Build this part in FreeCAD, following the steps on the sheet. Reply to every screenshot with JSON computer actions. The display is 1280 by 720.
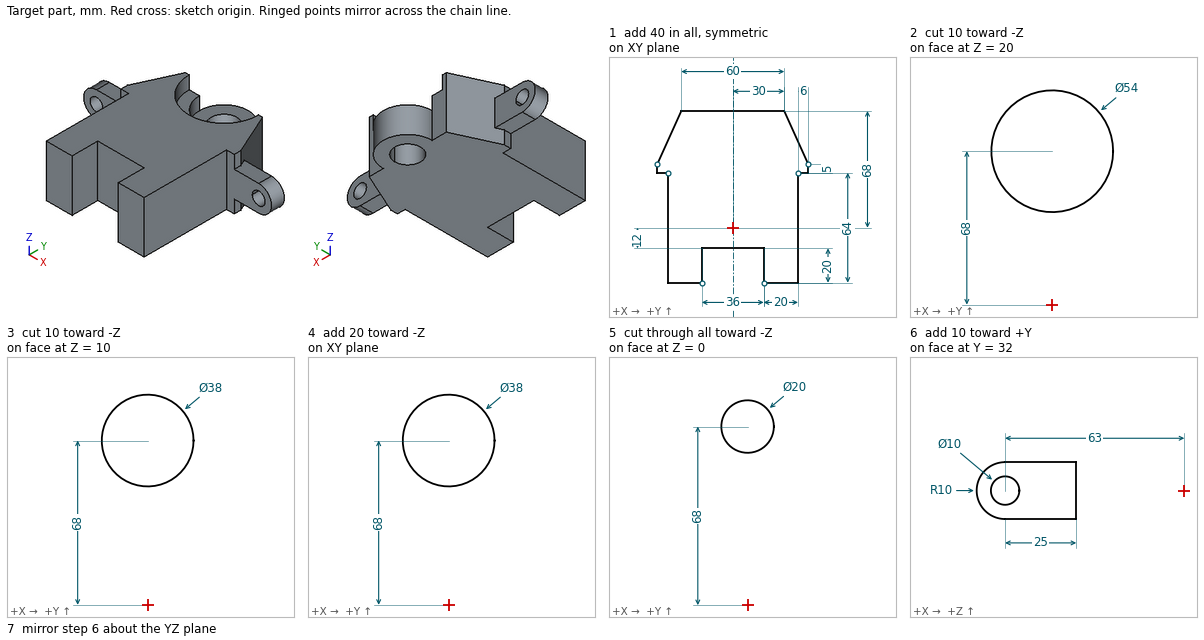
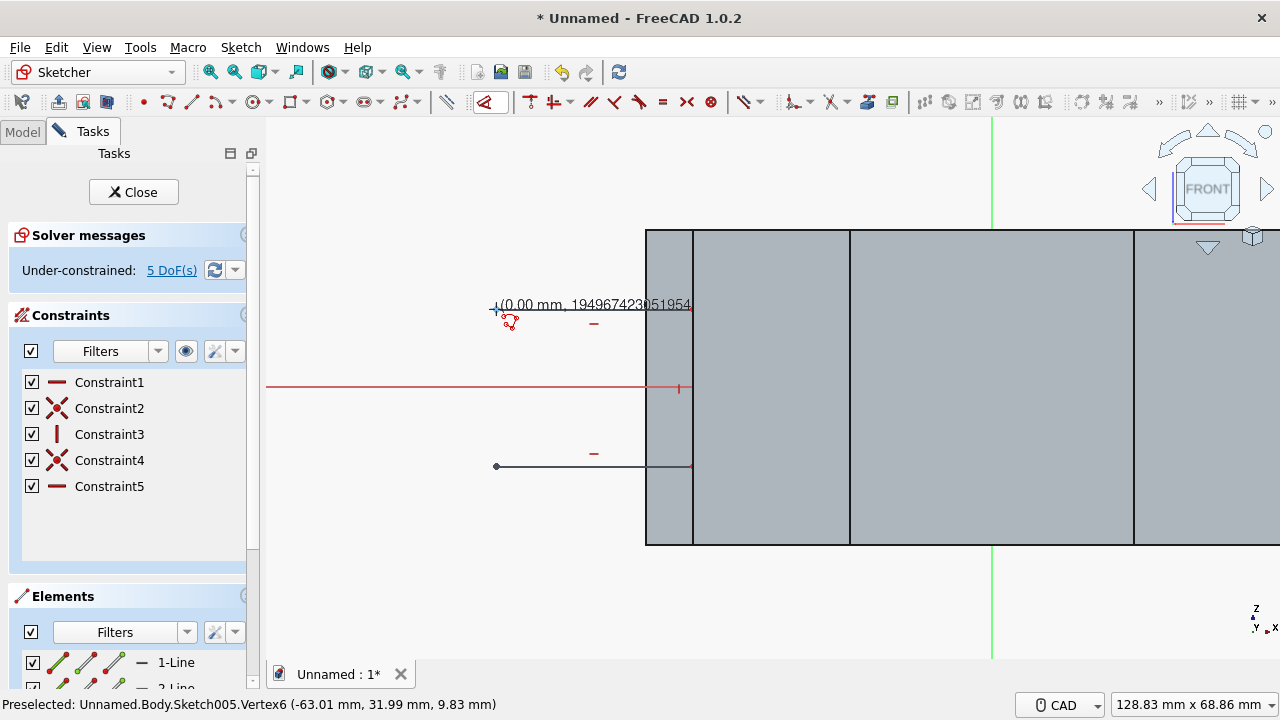
{"action": "key", "text": "g 3 a"}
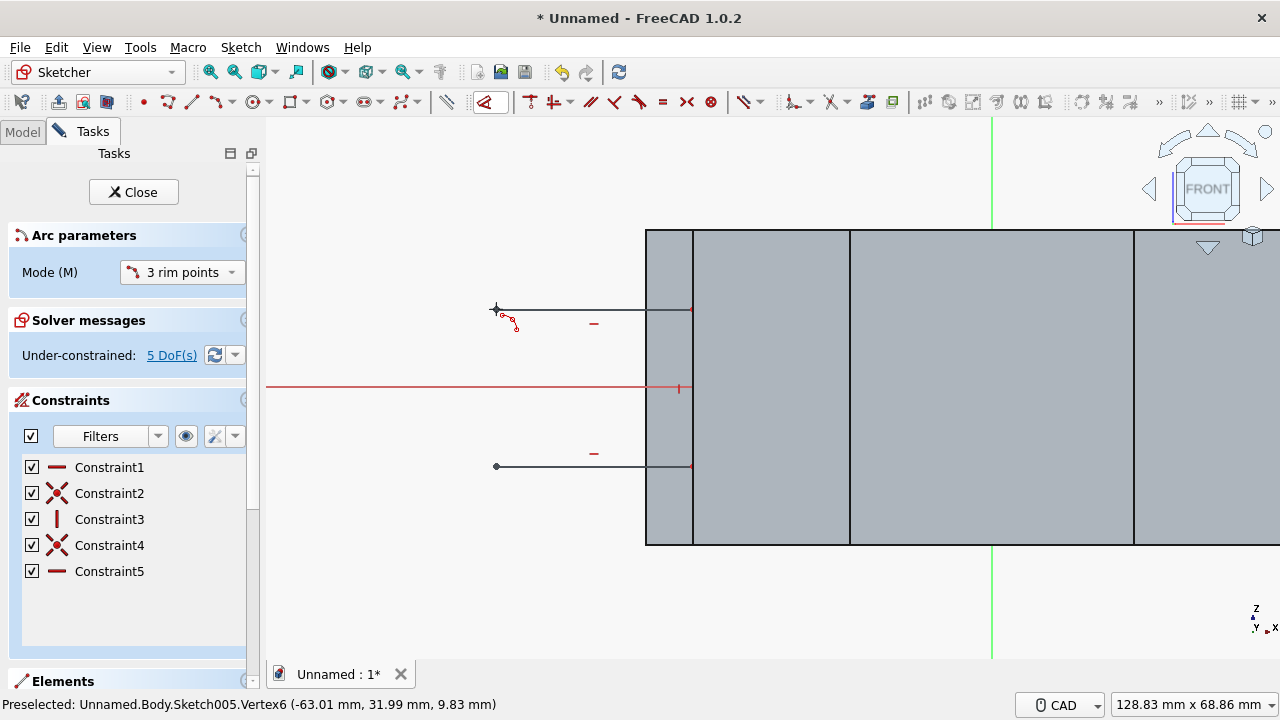
{"action": "left_click", "coordinate": [496, 310]}
{"action": "left_click", "coordinate": [496, 467]}
{"action": "left_click", "coordinate": [421, 363]}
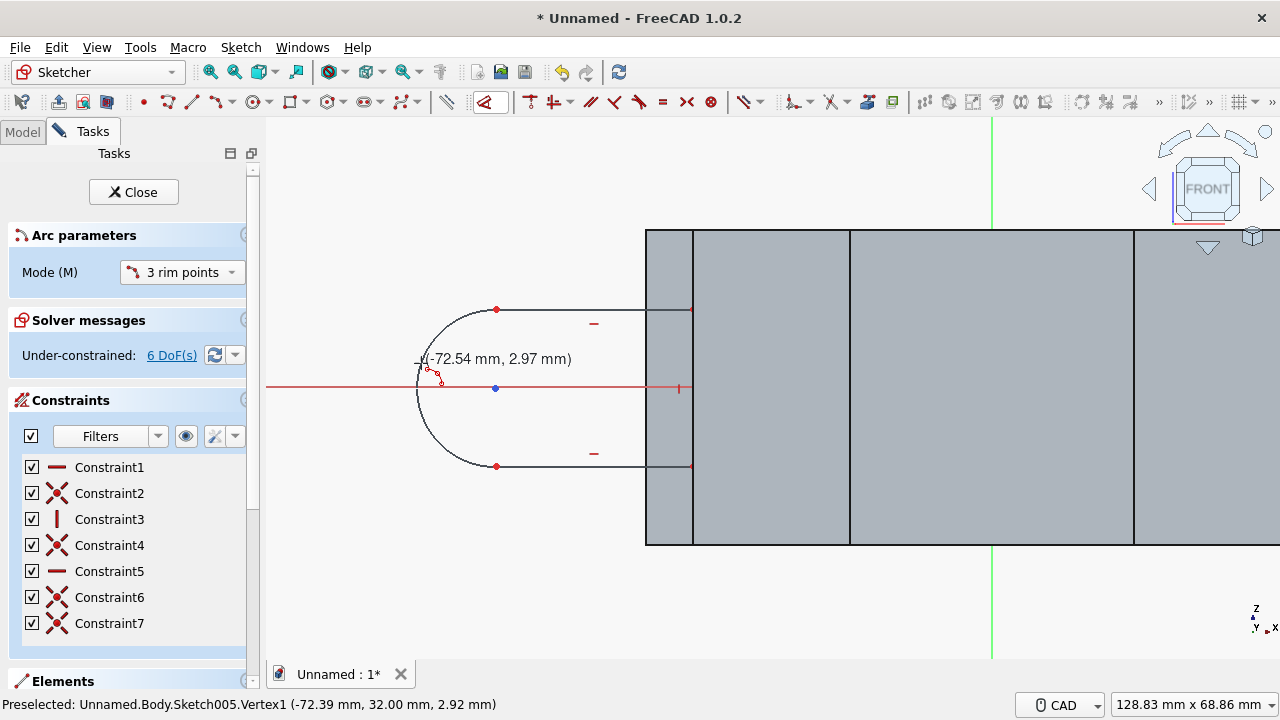
{"action": "left_click", "coordinate": [254, 102]}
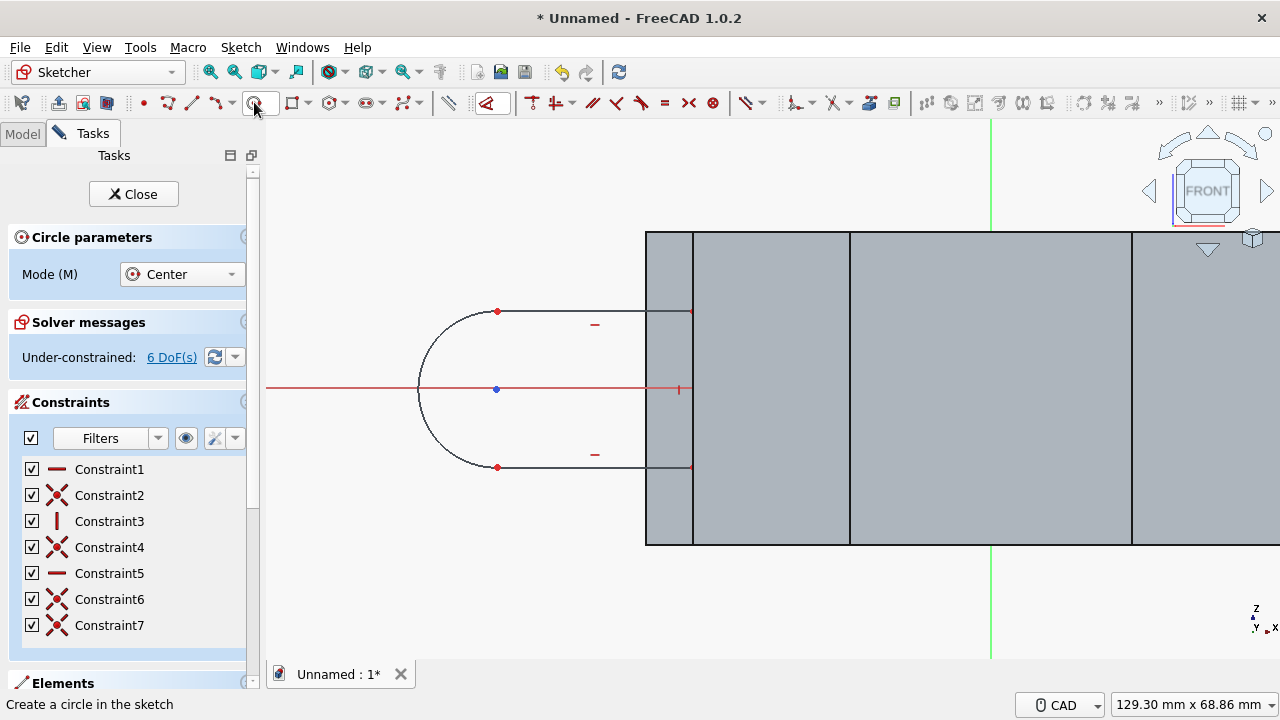
{"action": "left_click", "coordinate": [497, 388]}
{"action": "left_click", "coordinate": [525, 361]}
{"action": "key", "text": "Escape"}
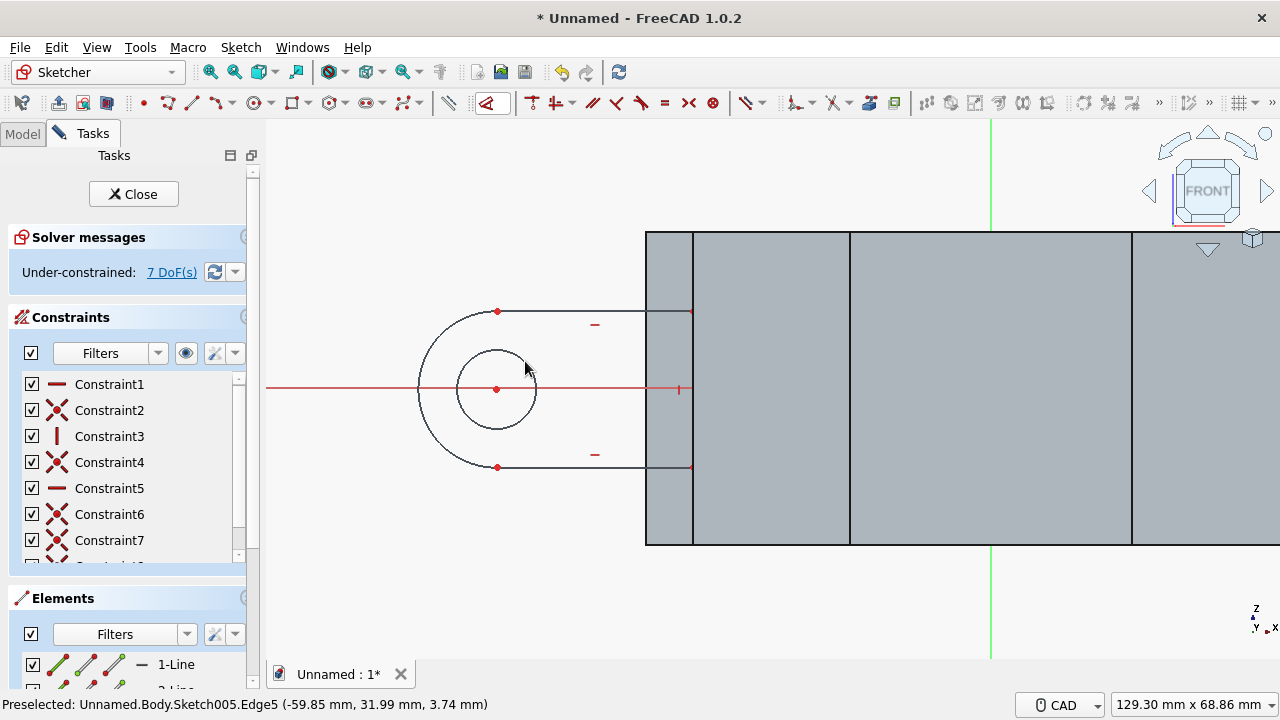
{"action": "left_click", "coordinate": [556, 468]}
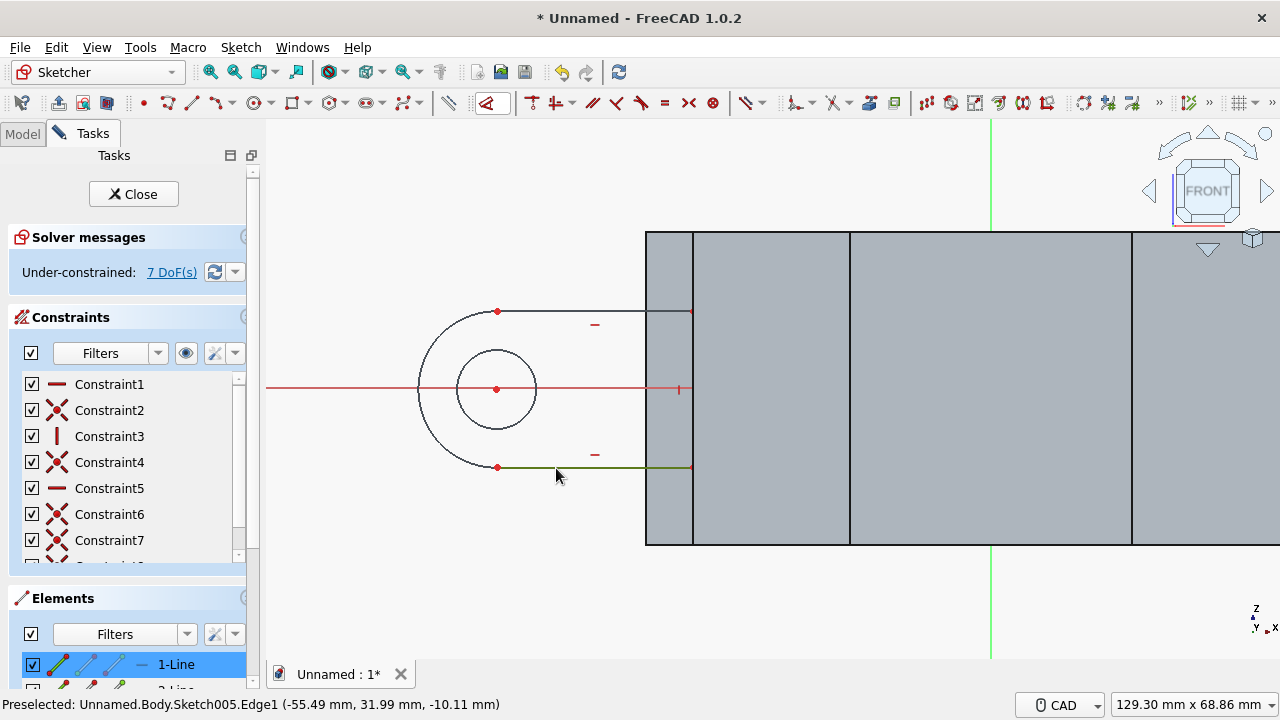
{"action": "left_click", "coordinate": [433, 343]}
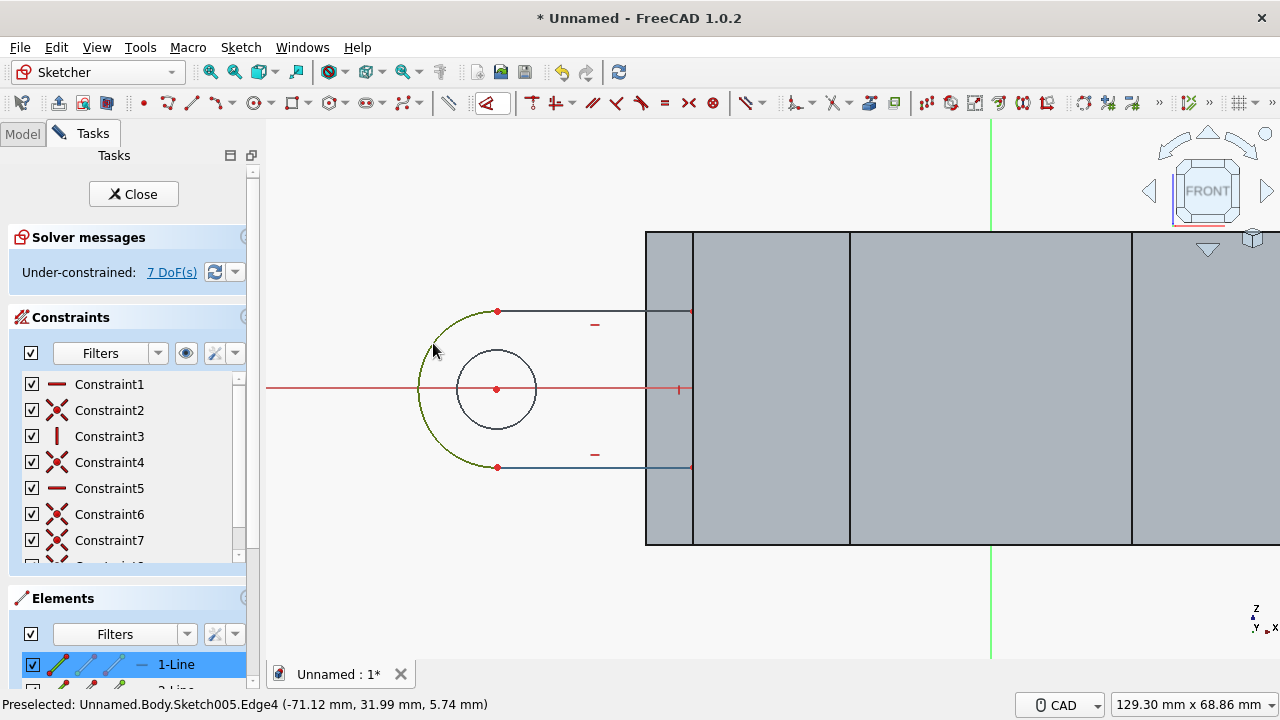
{"action": "left_click", "coordinate": [642, 104]}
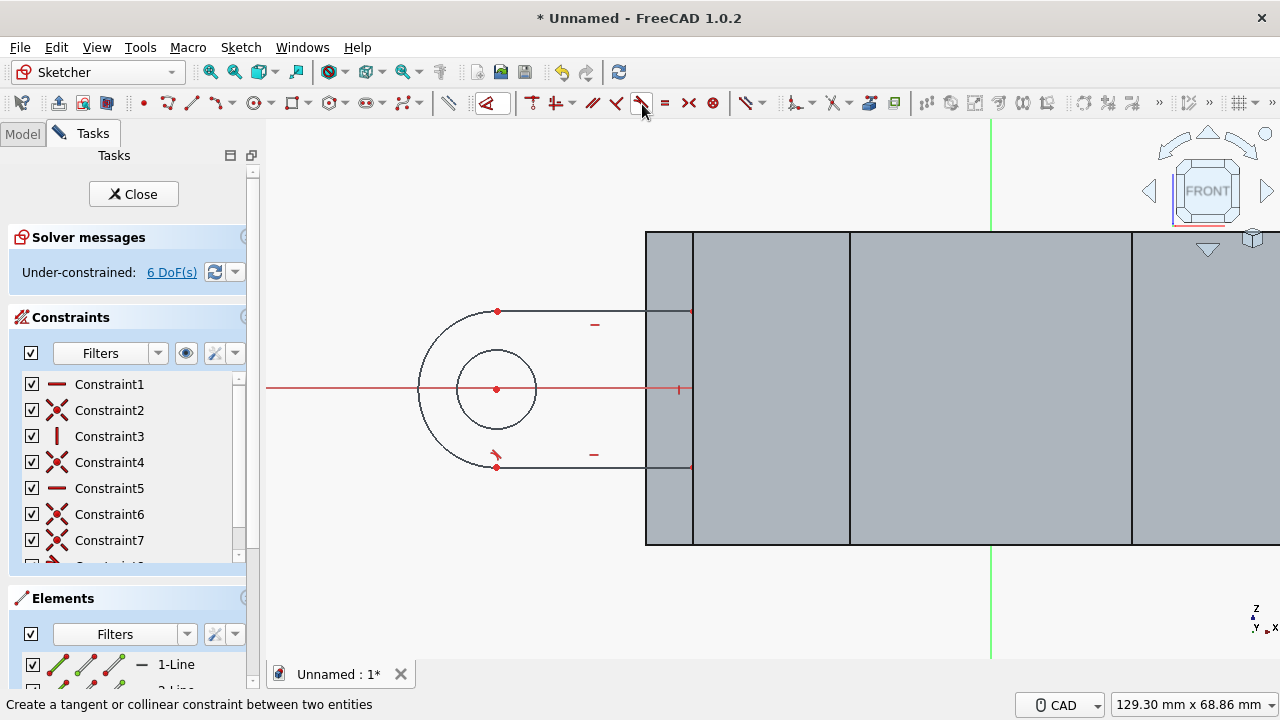
{"action": "left_click", "coordinate": [634, 311]}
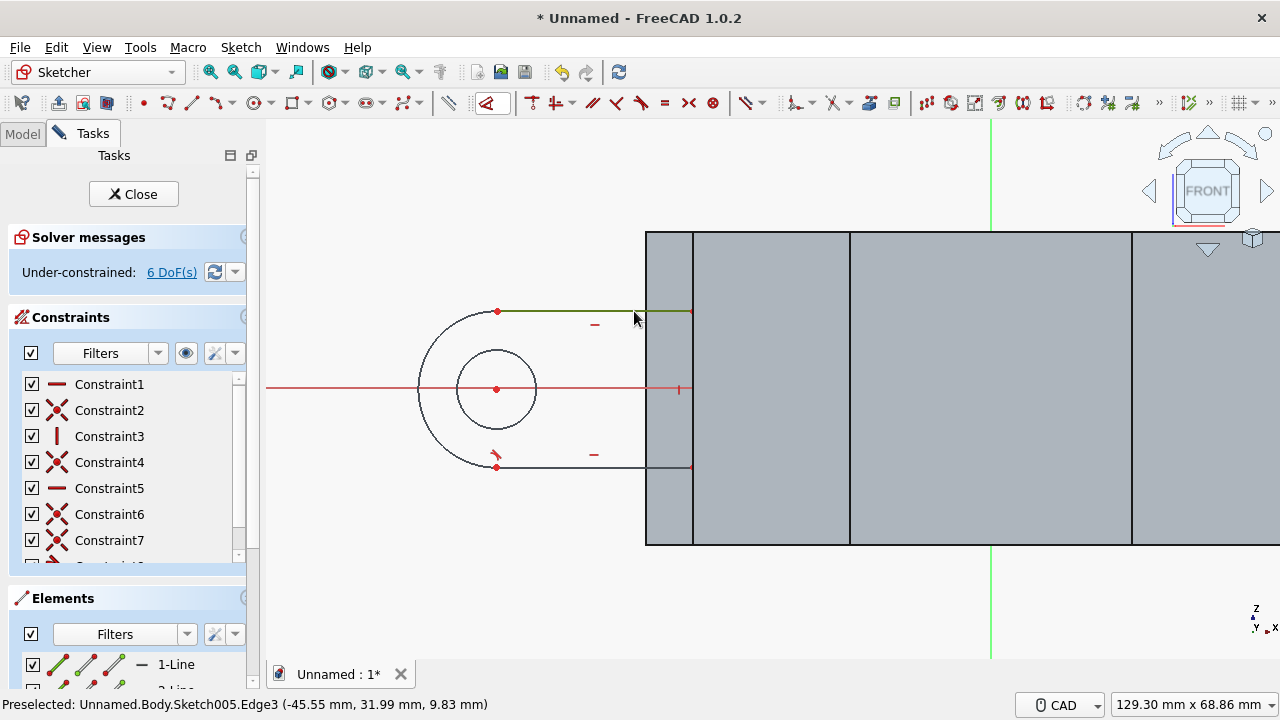
{"action": "left_click", "coordinate": [434, 343]}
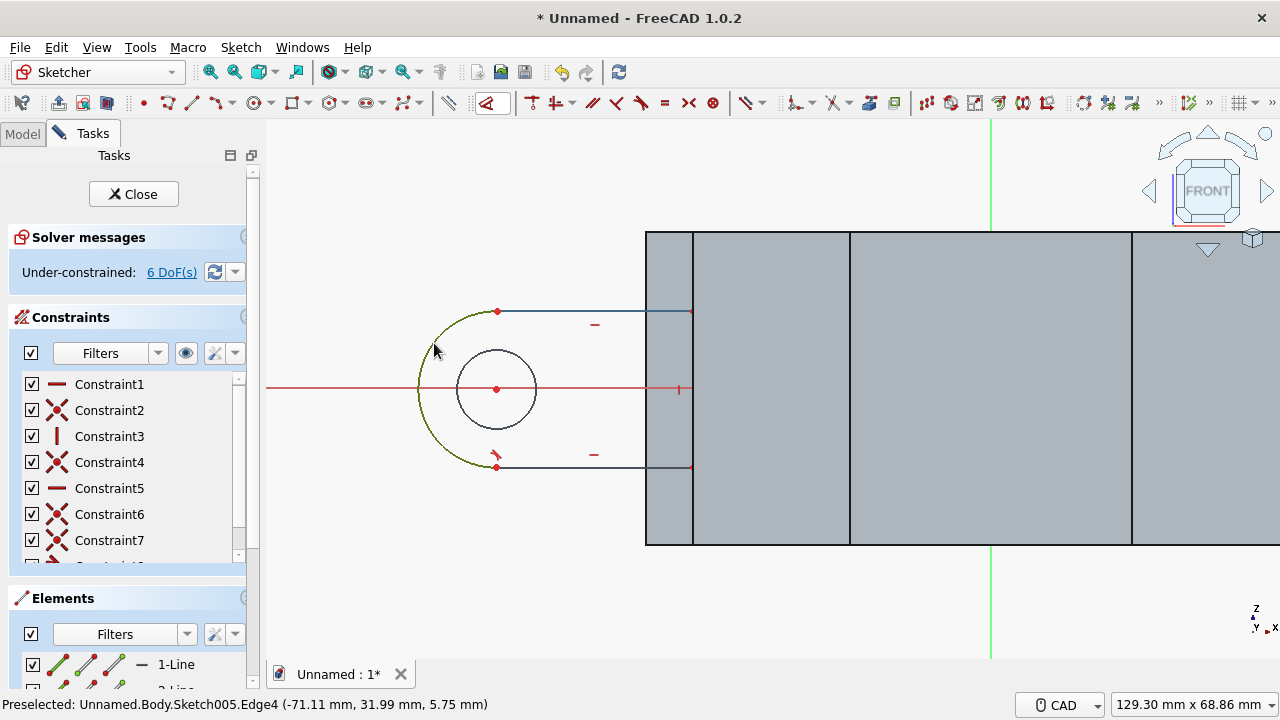
{"action": "left_click", "coordinate": [642, 104]}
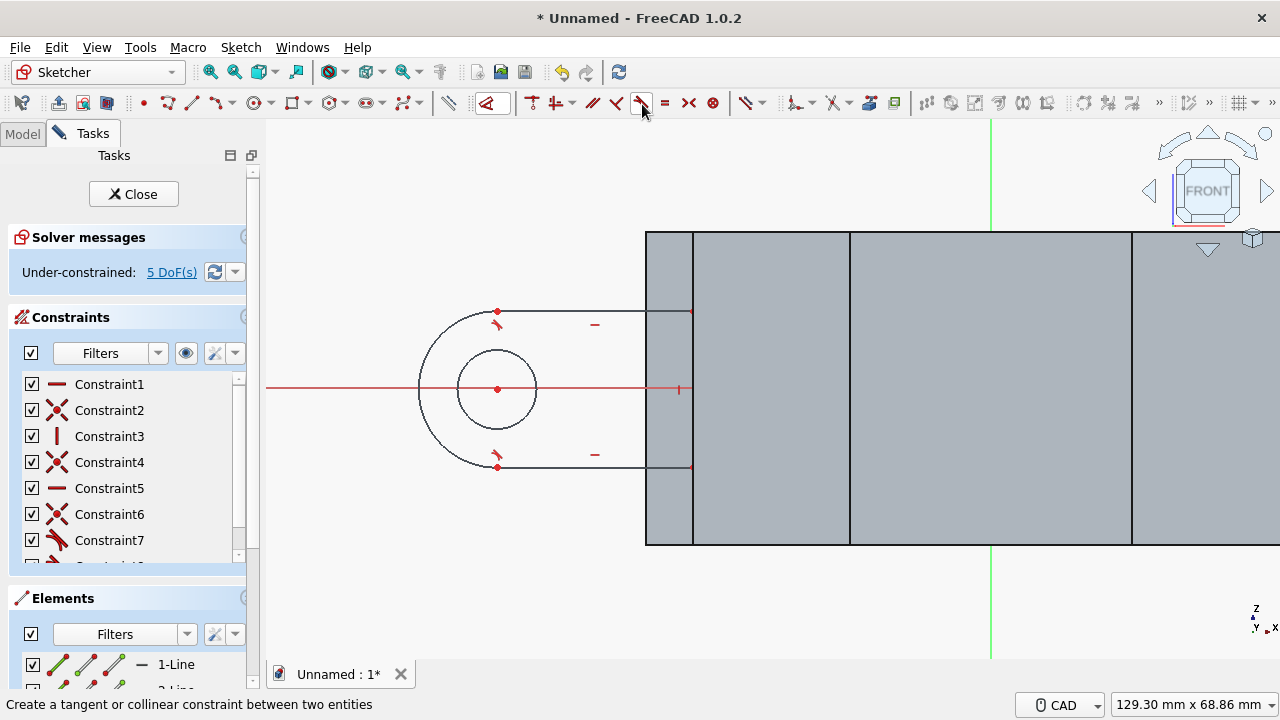
{"action": "left_click", "coordinate": [497, 389]}